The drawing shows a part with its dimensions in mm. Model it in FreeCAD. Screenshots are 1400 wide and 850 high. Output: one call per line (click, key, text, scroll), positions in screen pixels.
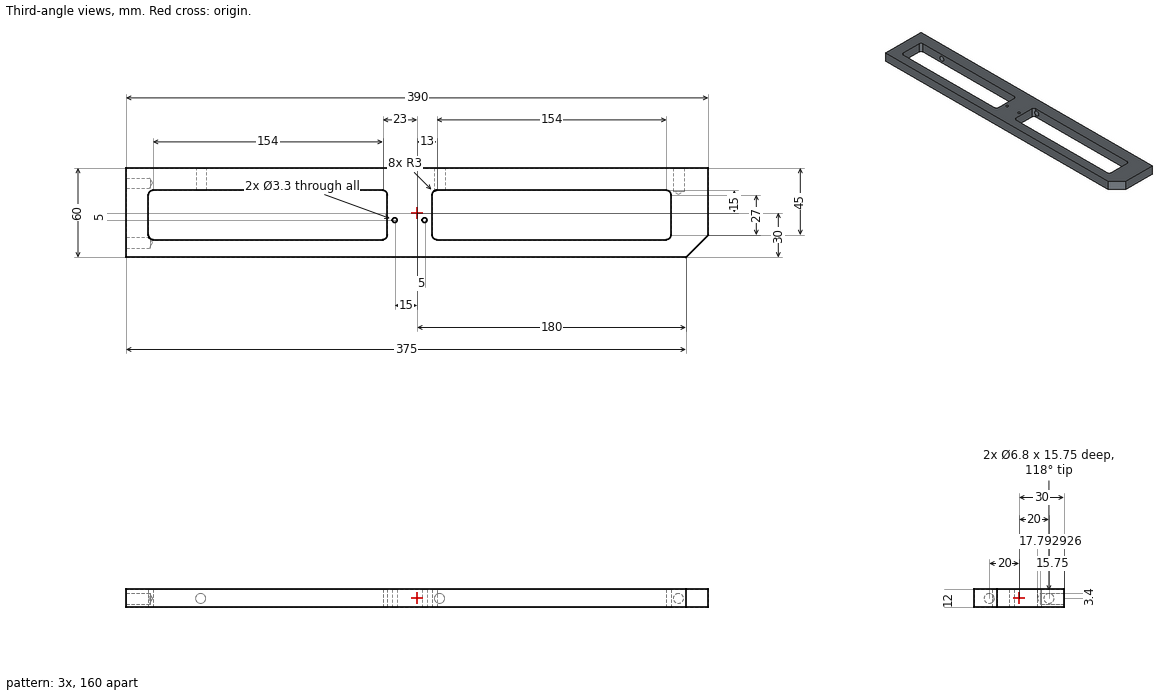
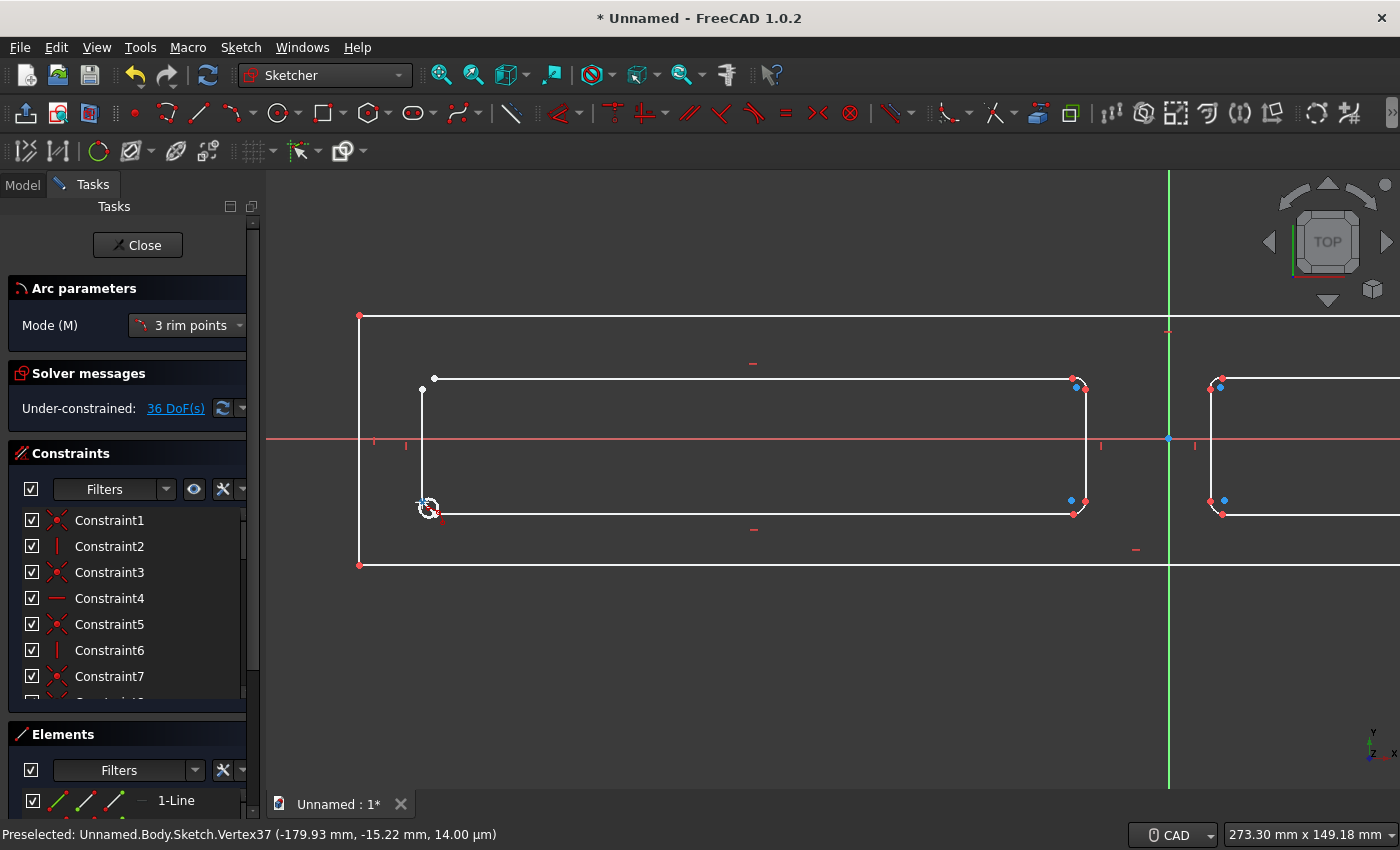
scroll(426, 510, up, 8)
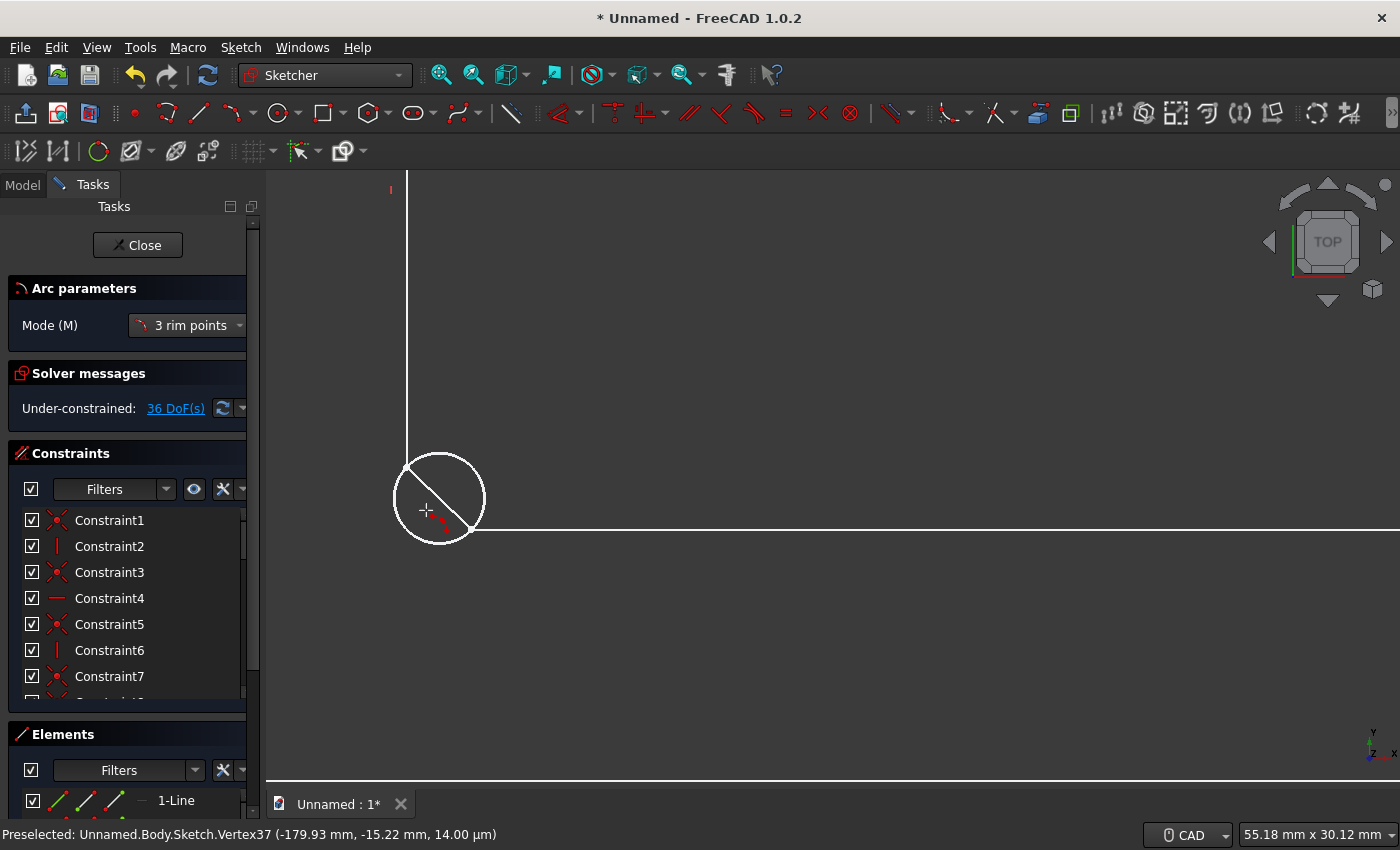
click(423, 506)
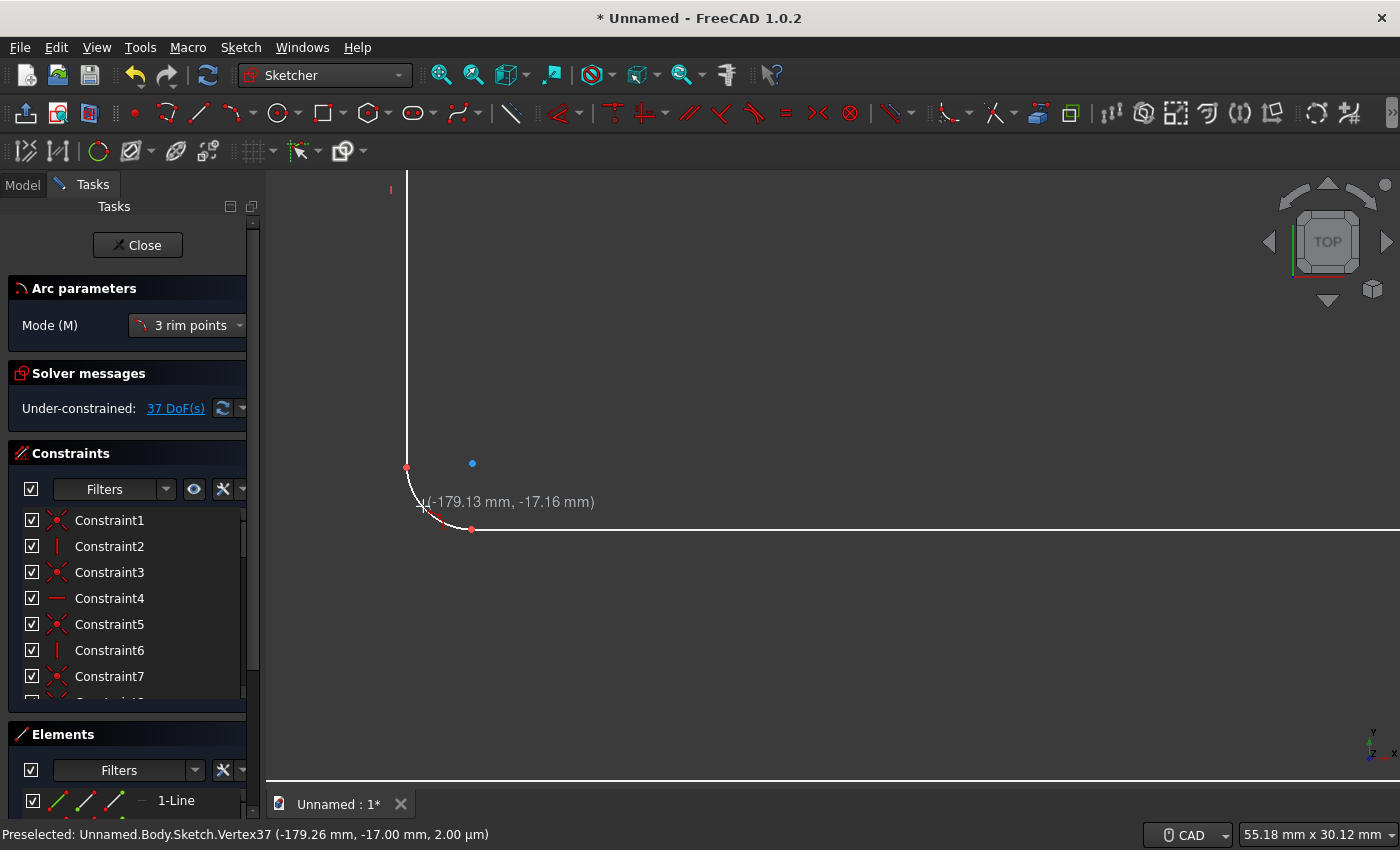
scroll(431, 512, down, 12)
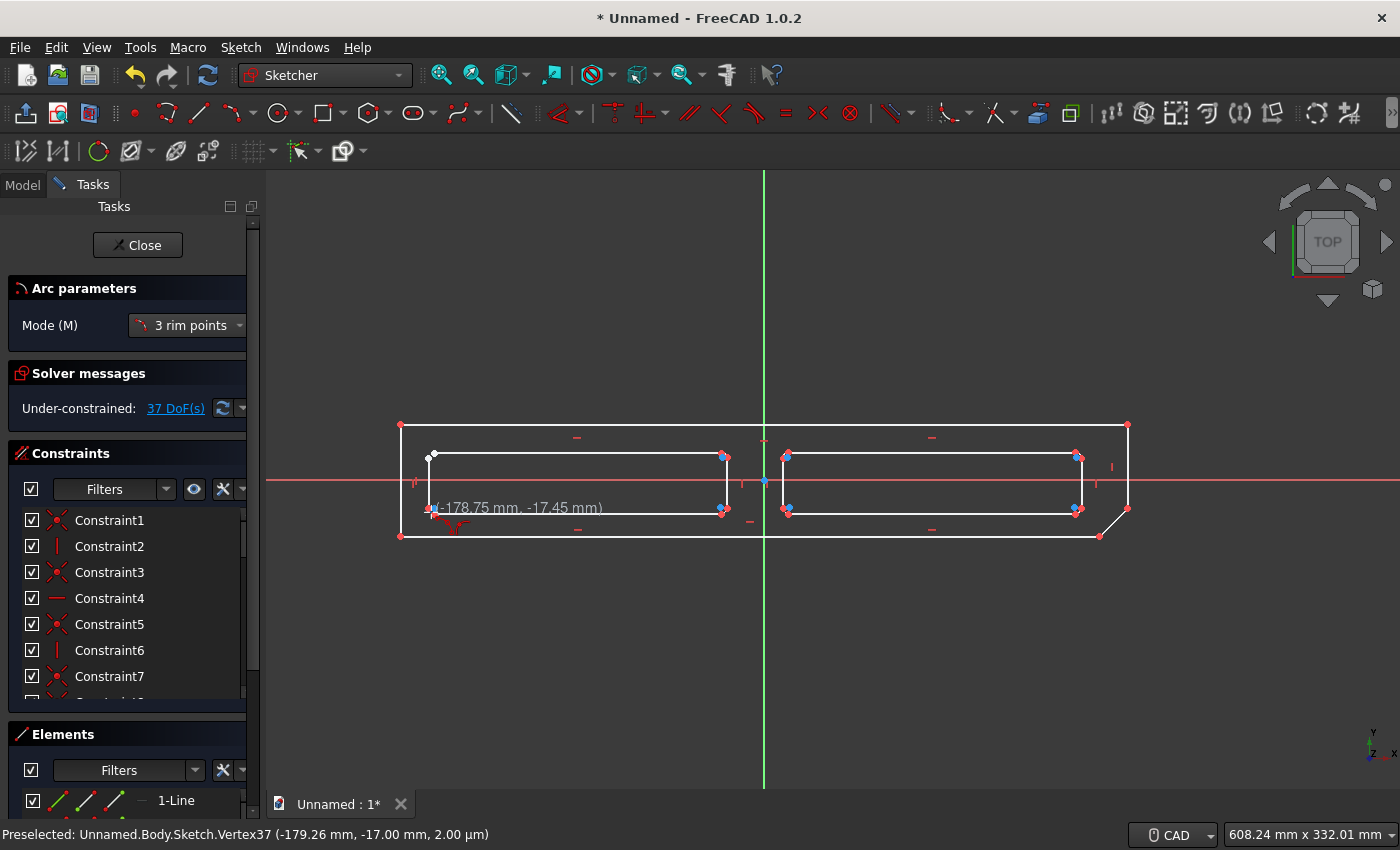
scroll(429, 458, up, 4)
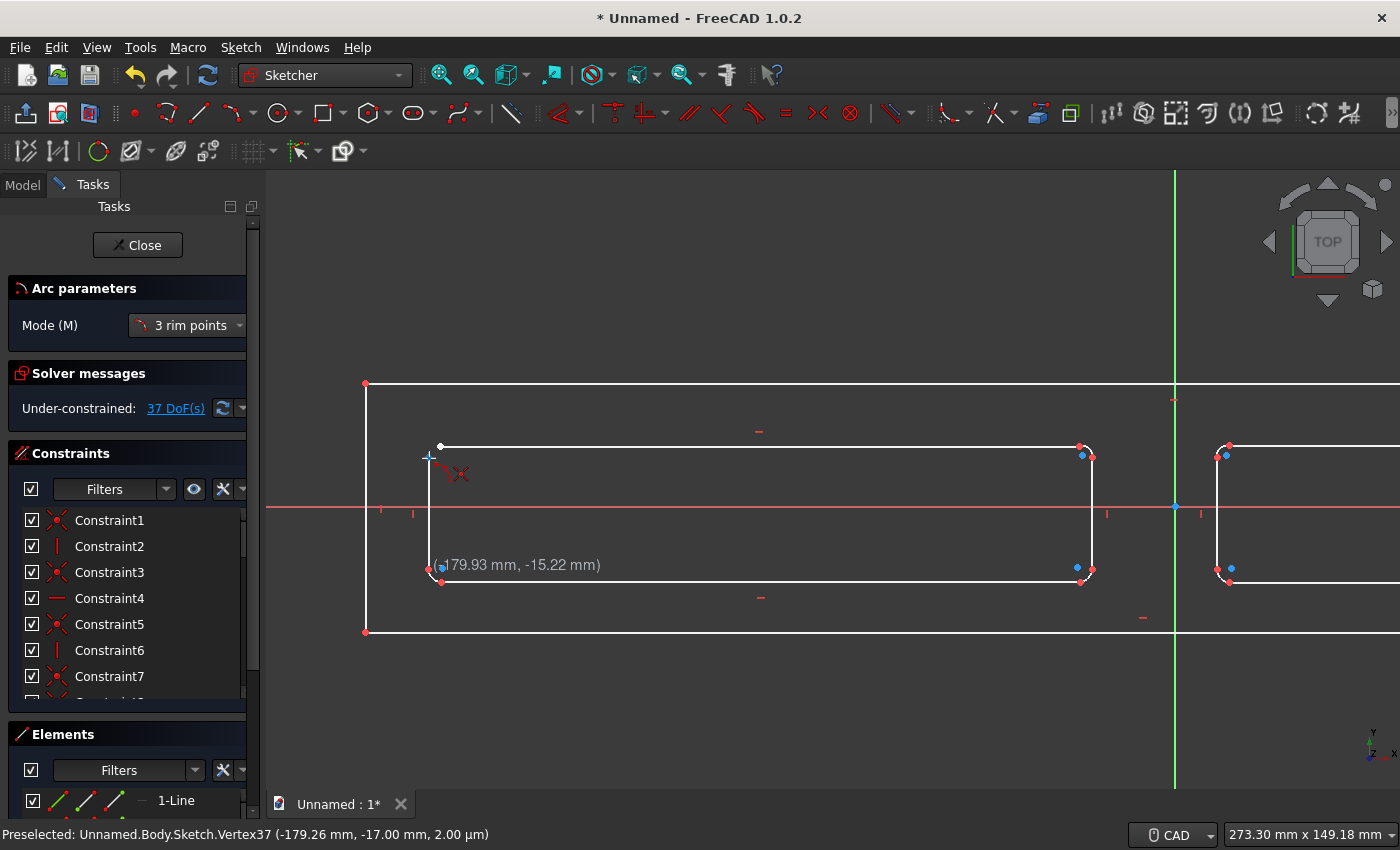
click(429, 458)
click(441, 447)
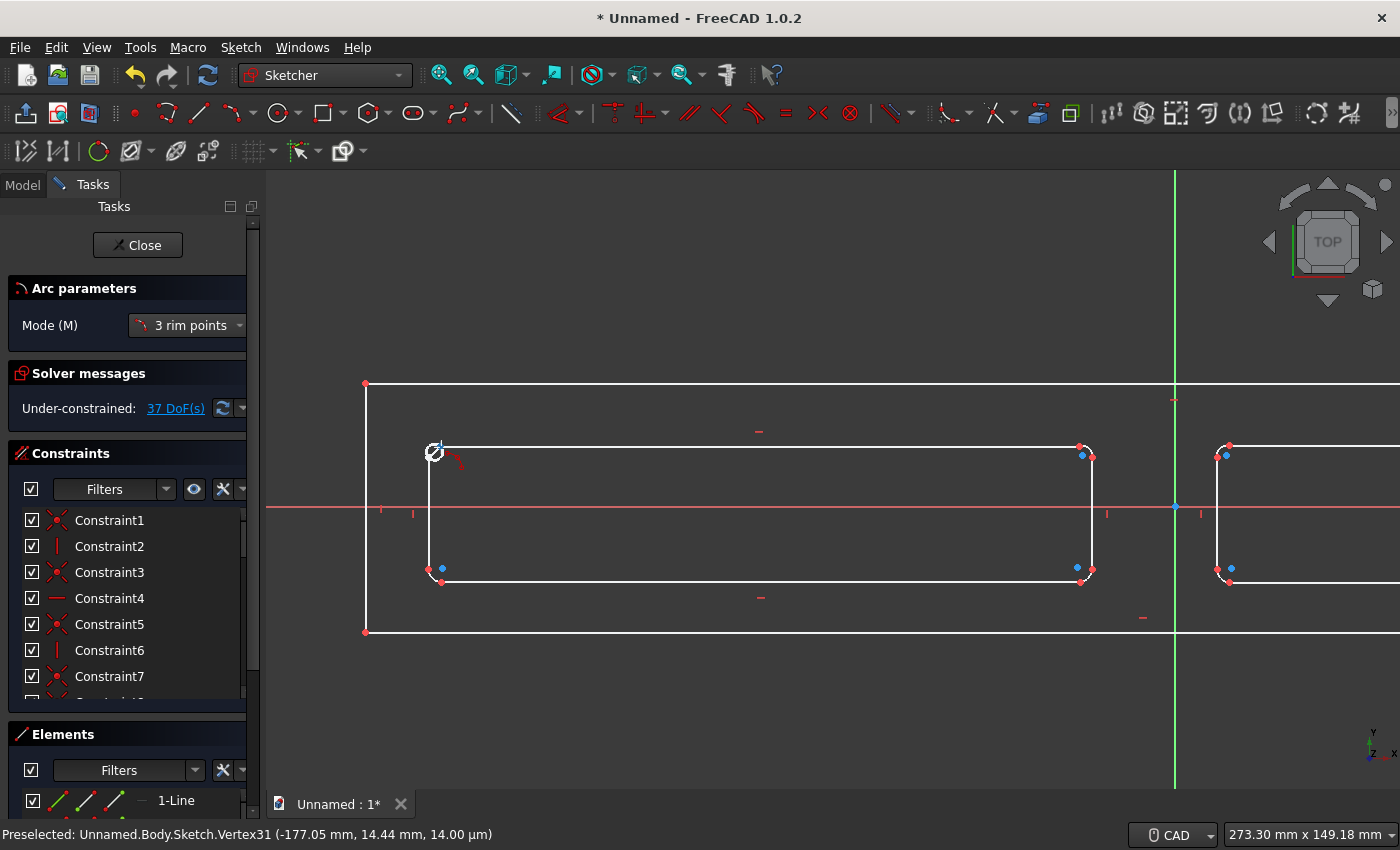
scroll(432, 448, up, 8)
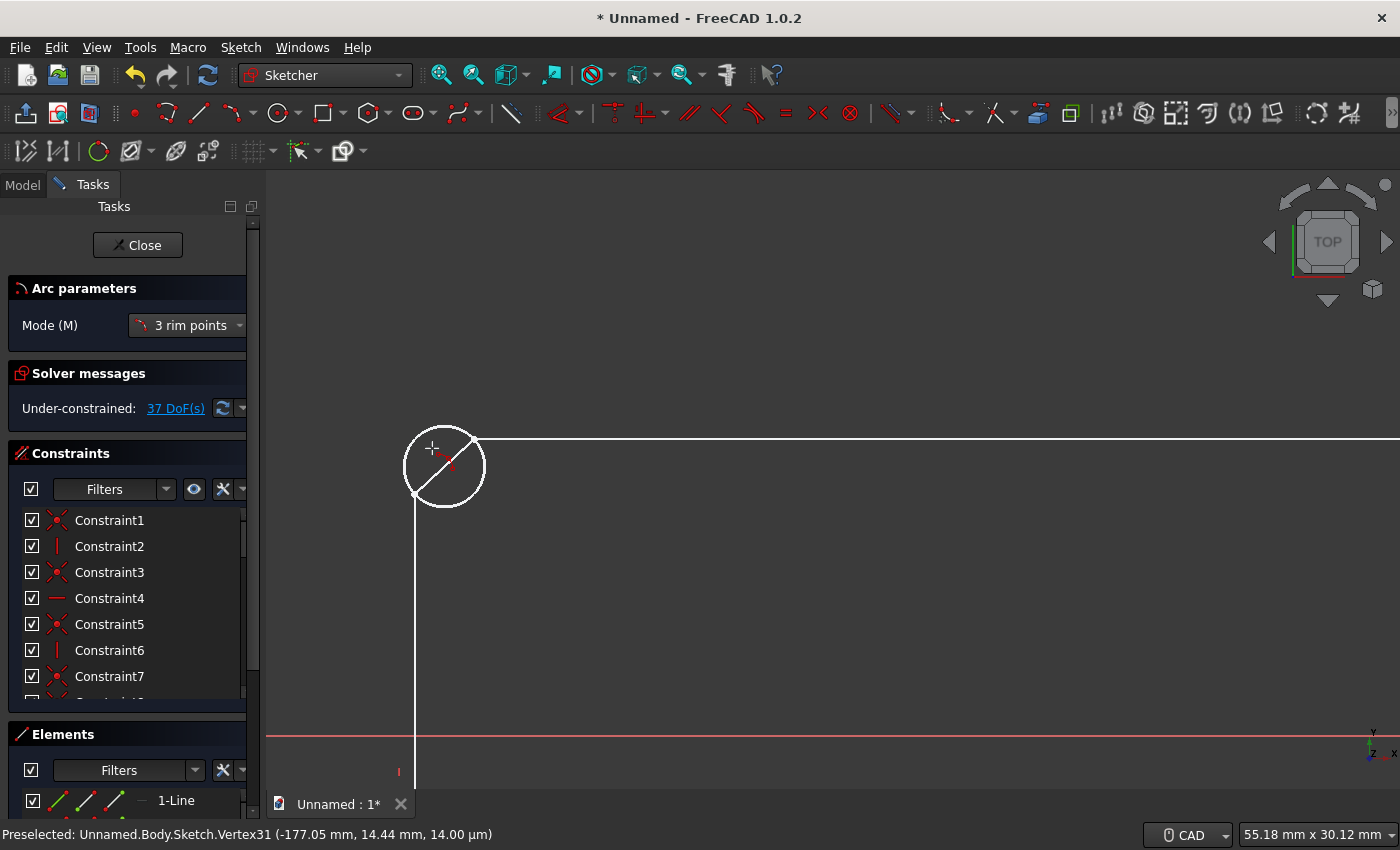
click(431, 446)
key(Escape)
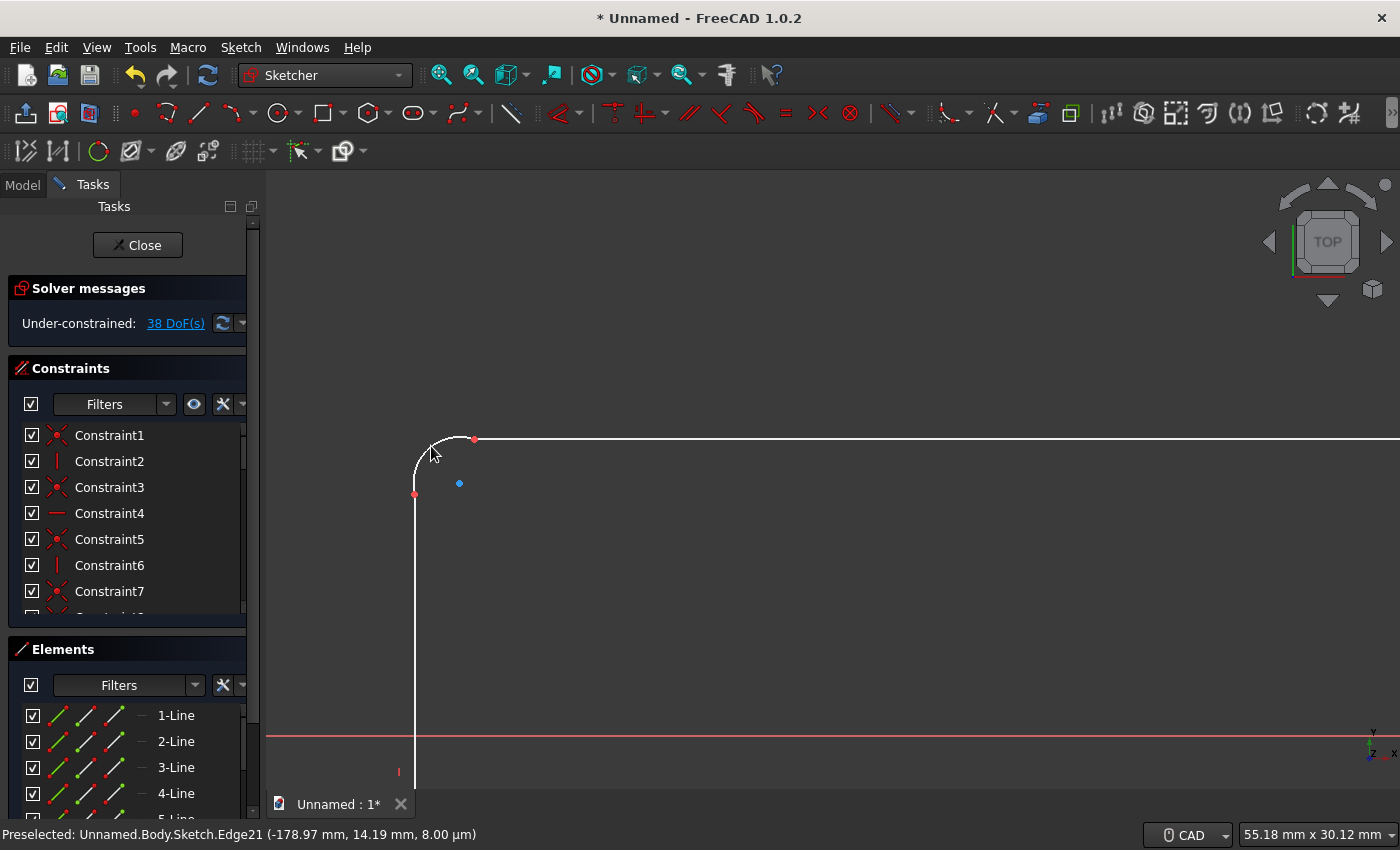
scroll(430, 454, down, 12)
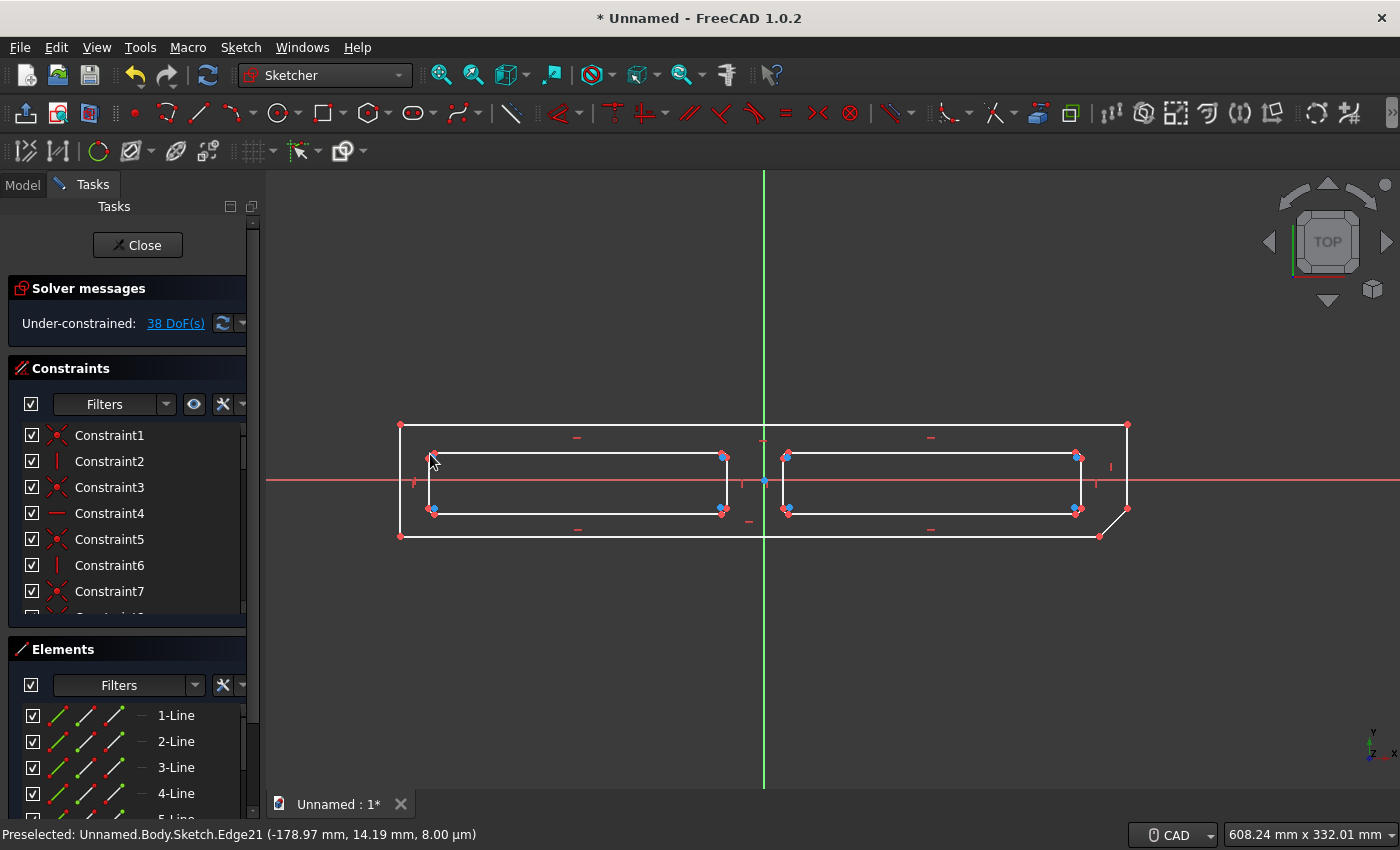
click(875, 453)